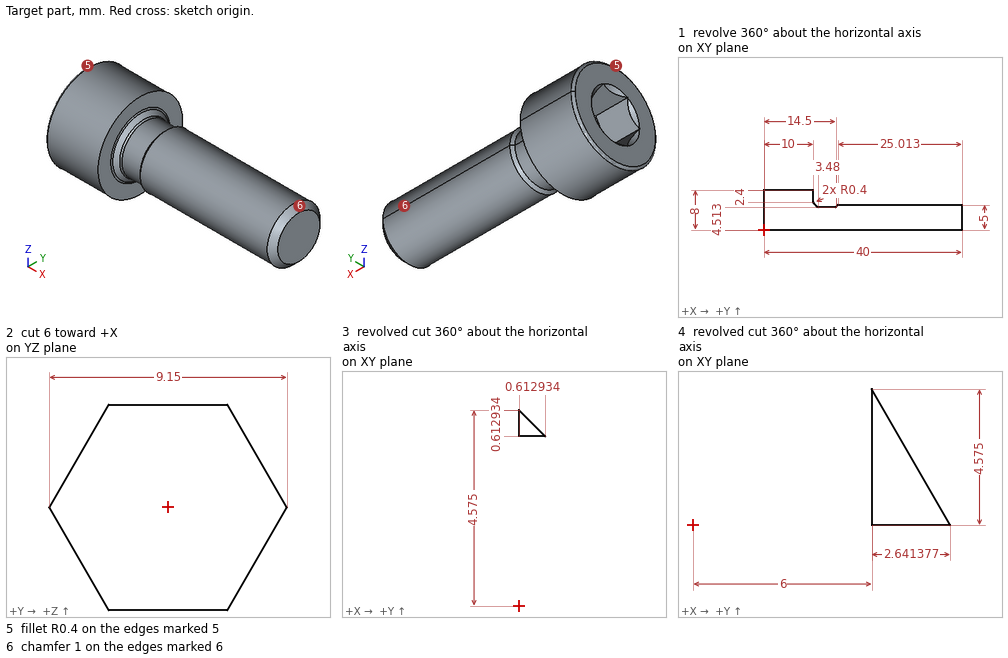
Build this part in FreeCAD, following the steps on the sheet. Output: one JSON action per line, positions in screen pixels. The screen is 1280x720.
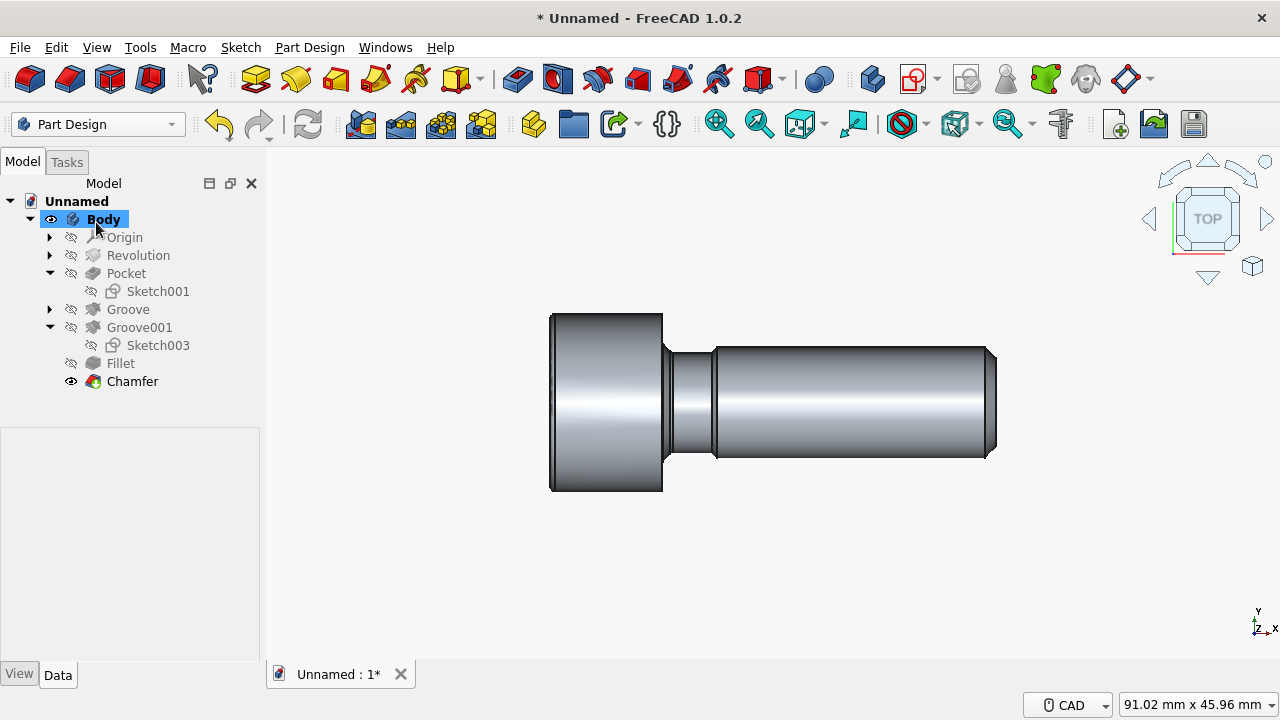
{"action": "key", "text": "0"}